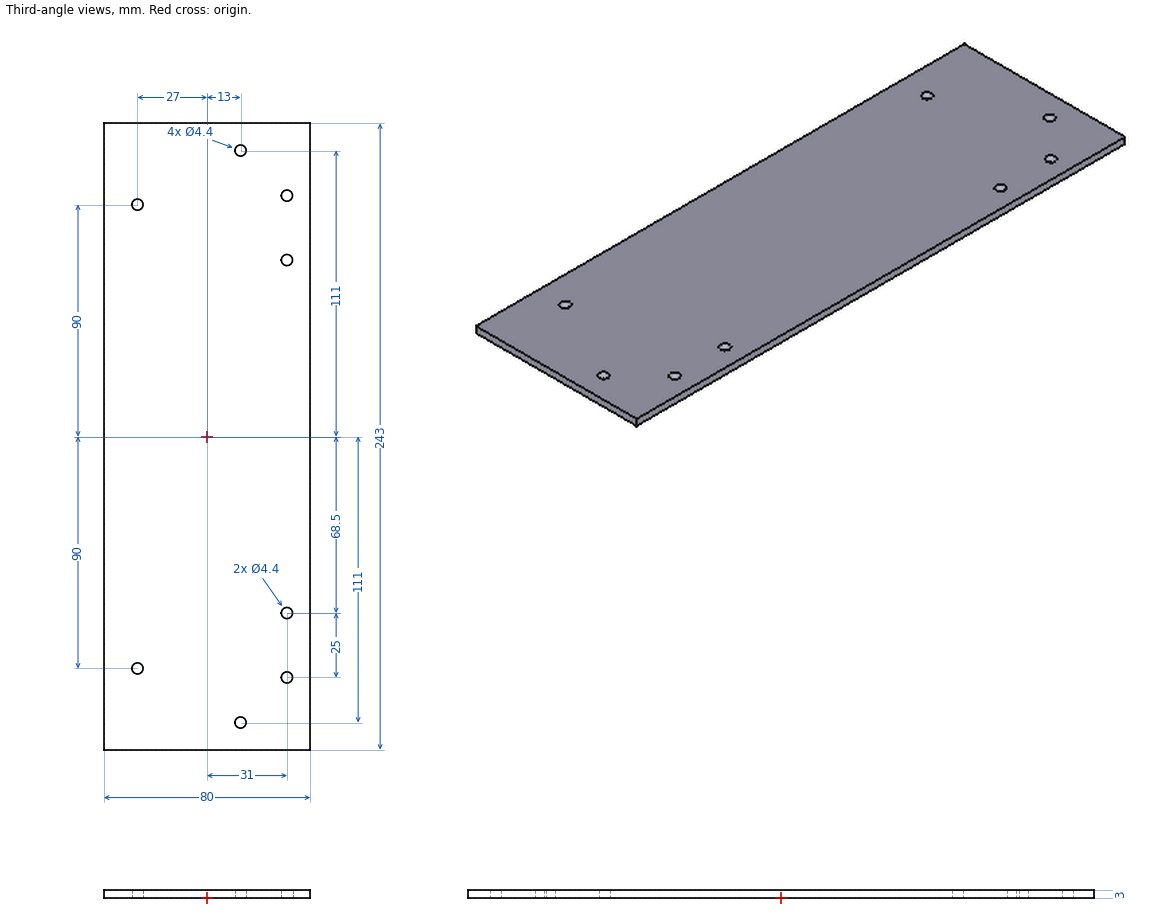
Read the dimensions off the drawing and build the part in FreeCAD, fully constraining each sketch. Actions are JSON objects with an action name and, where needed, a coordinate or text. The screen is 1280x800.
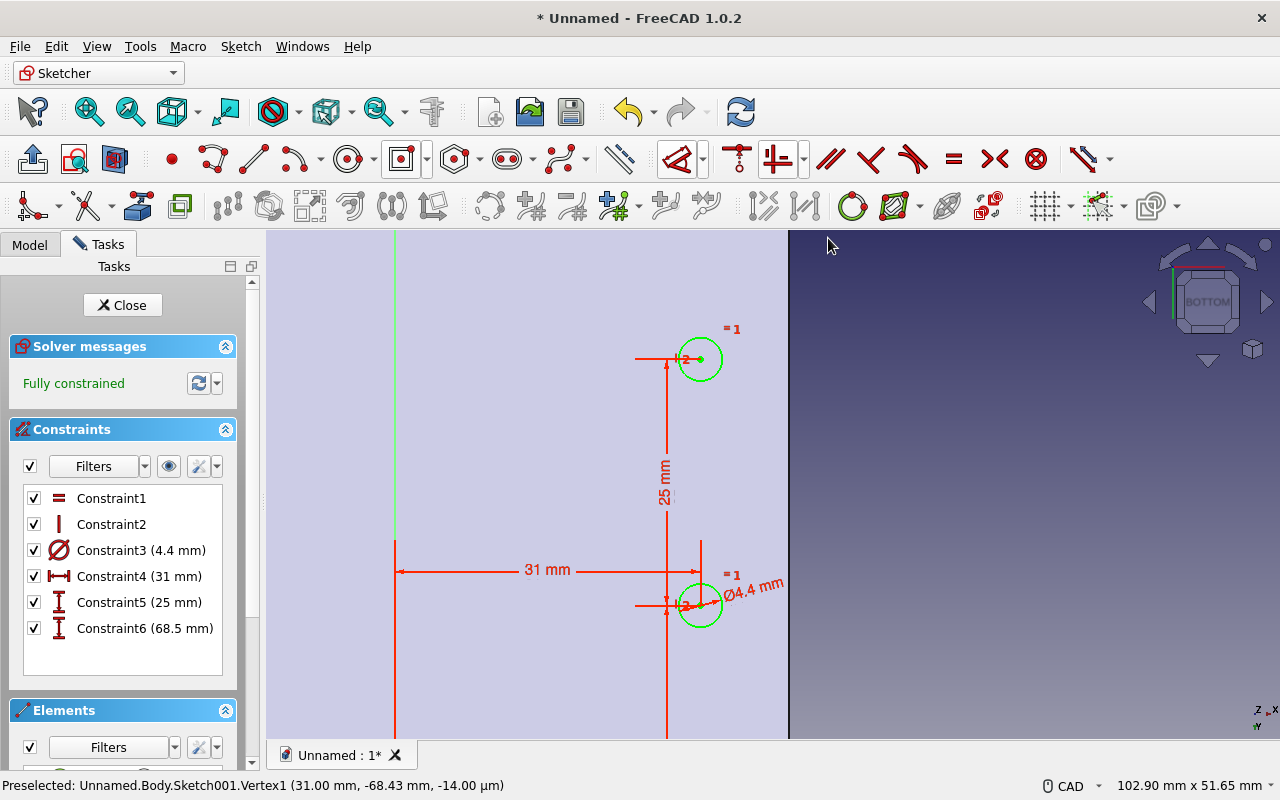
{"action": "left_click", "coordinate": [123, 305]}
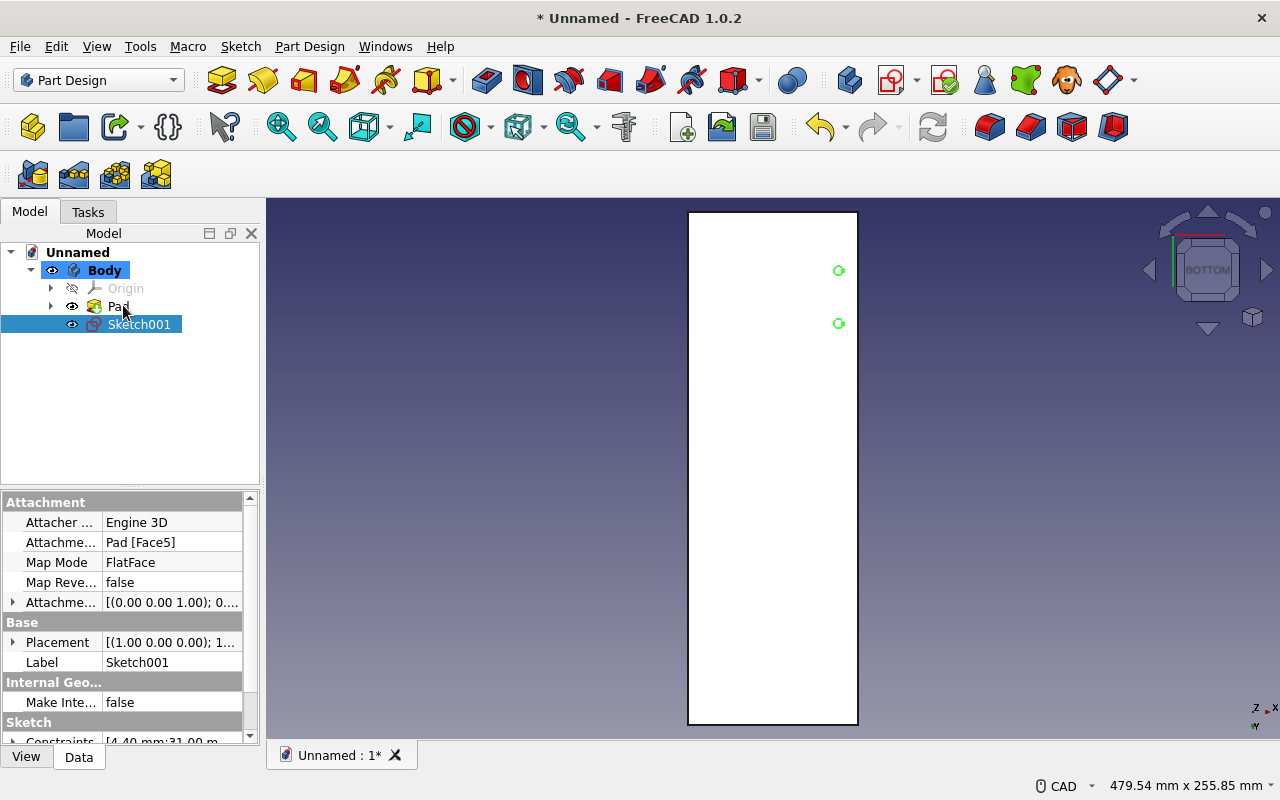
{"action": "left_click", "coordinate": [487, 80]}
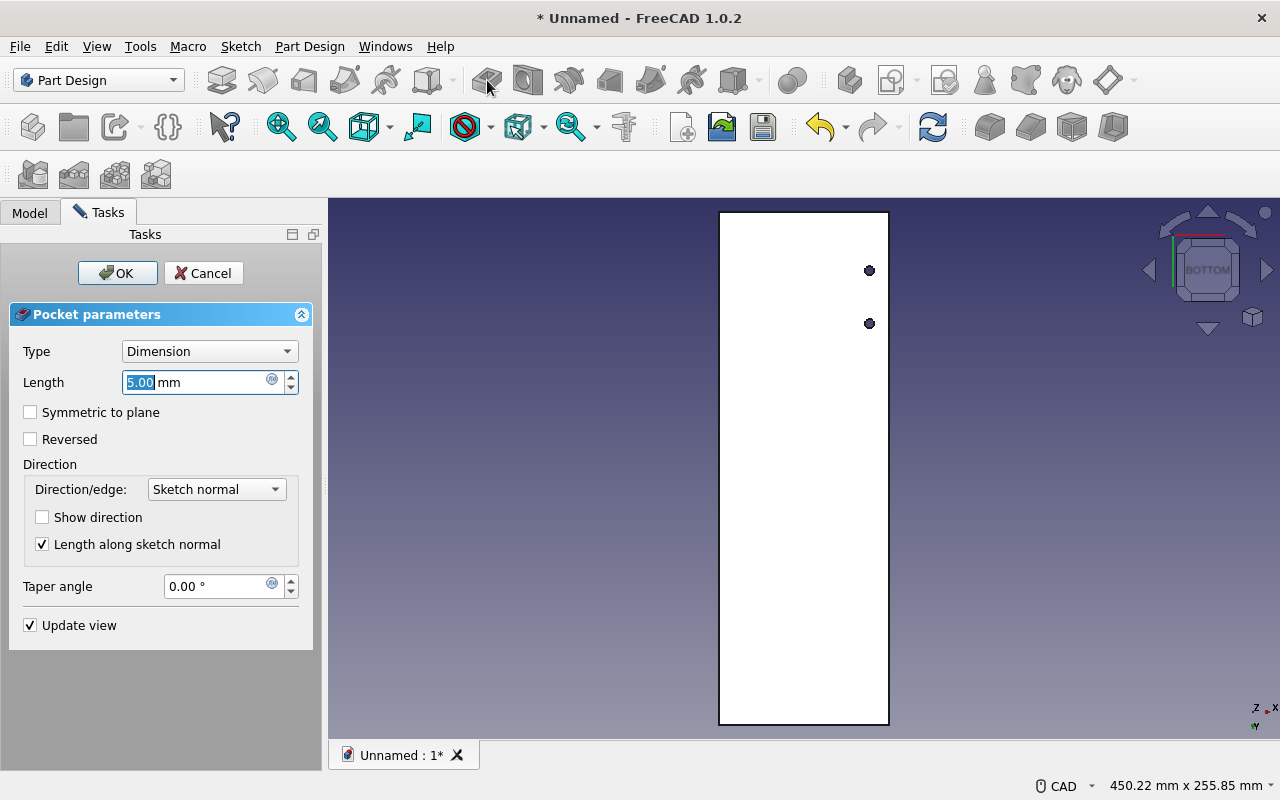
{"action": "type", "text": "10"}
{"action": "key", "text": "Tab"}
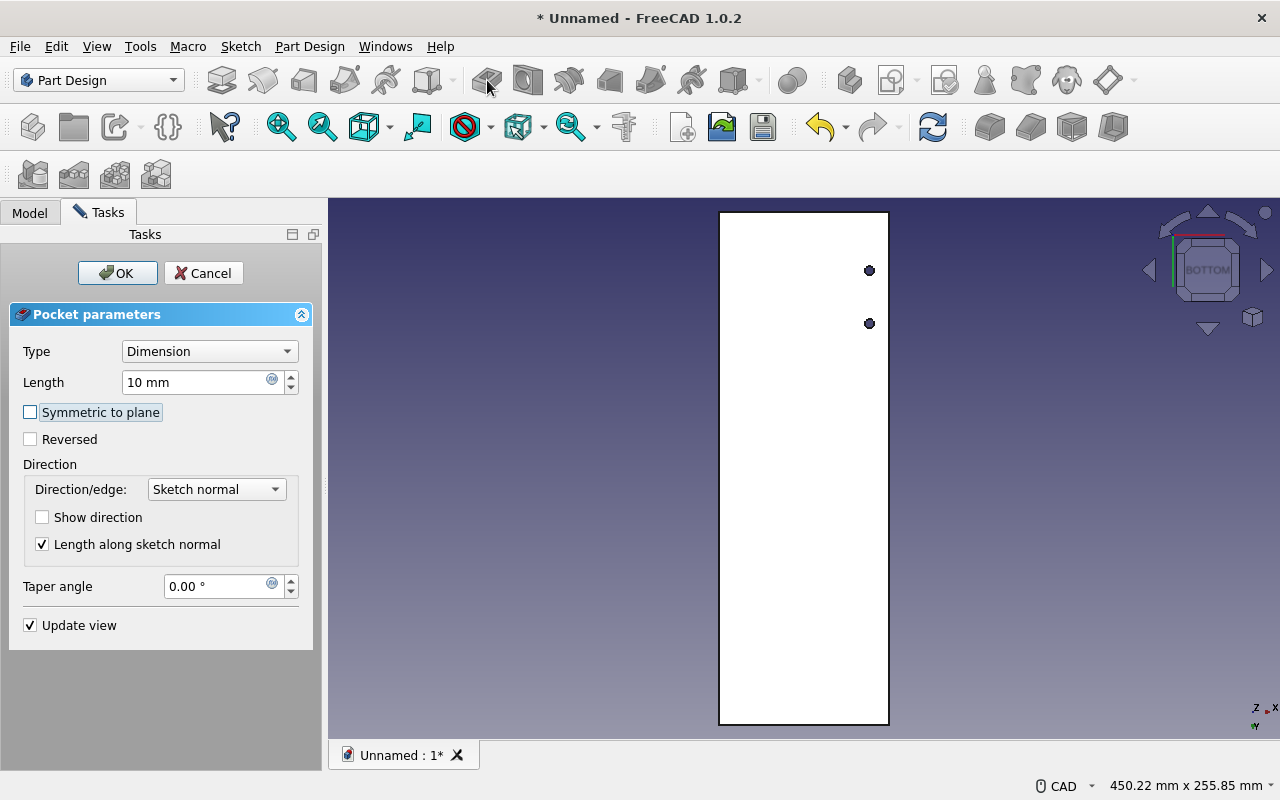
{"action": "left_click", "coordinate": [118, 273]}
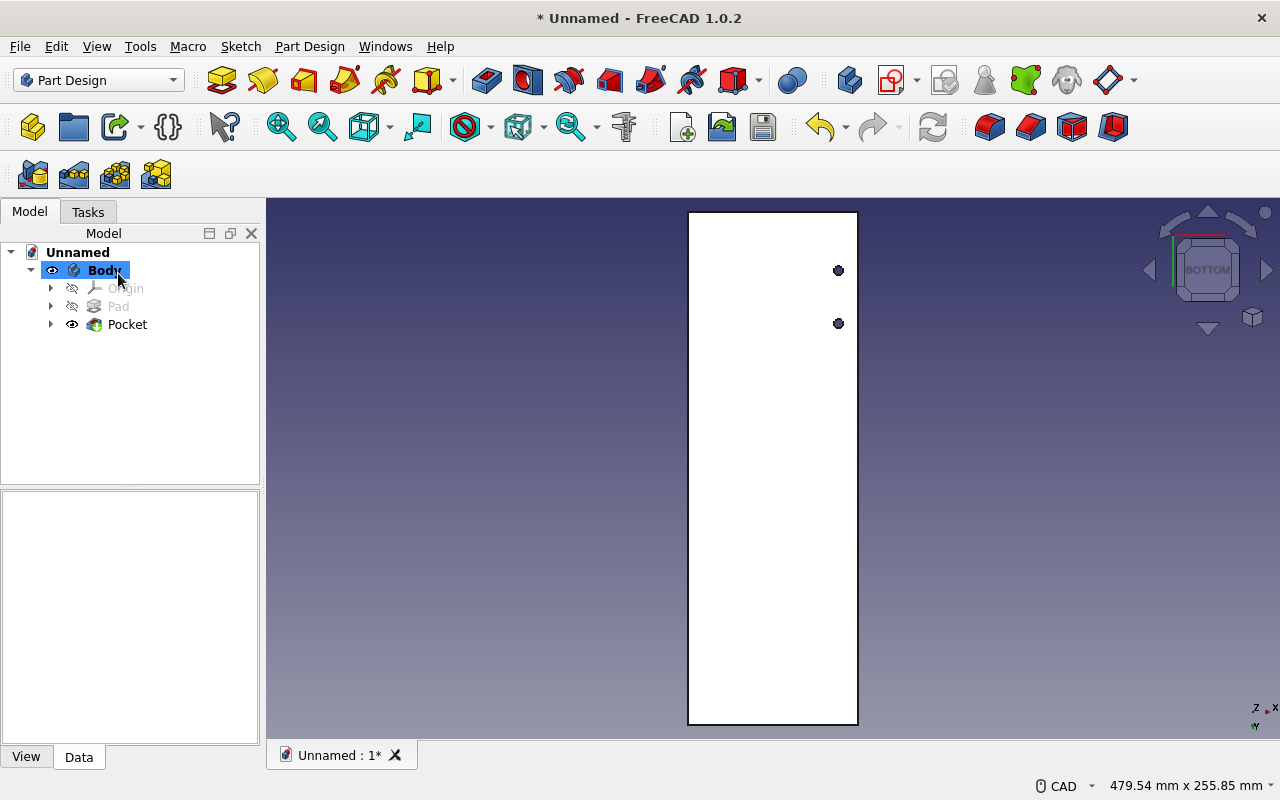
{"action": "left_click", "coordinate": [117, 324]}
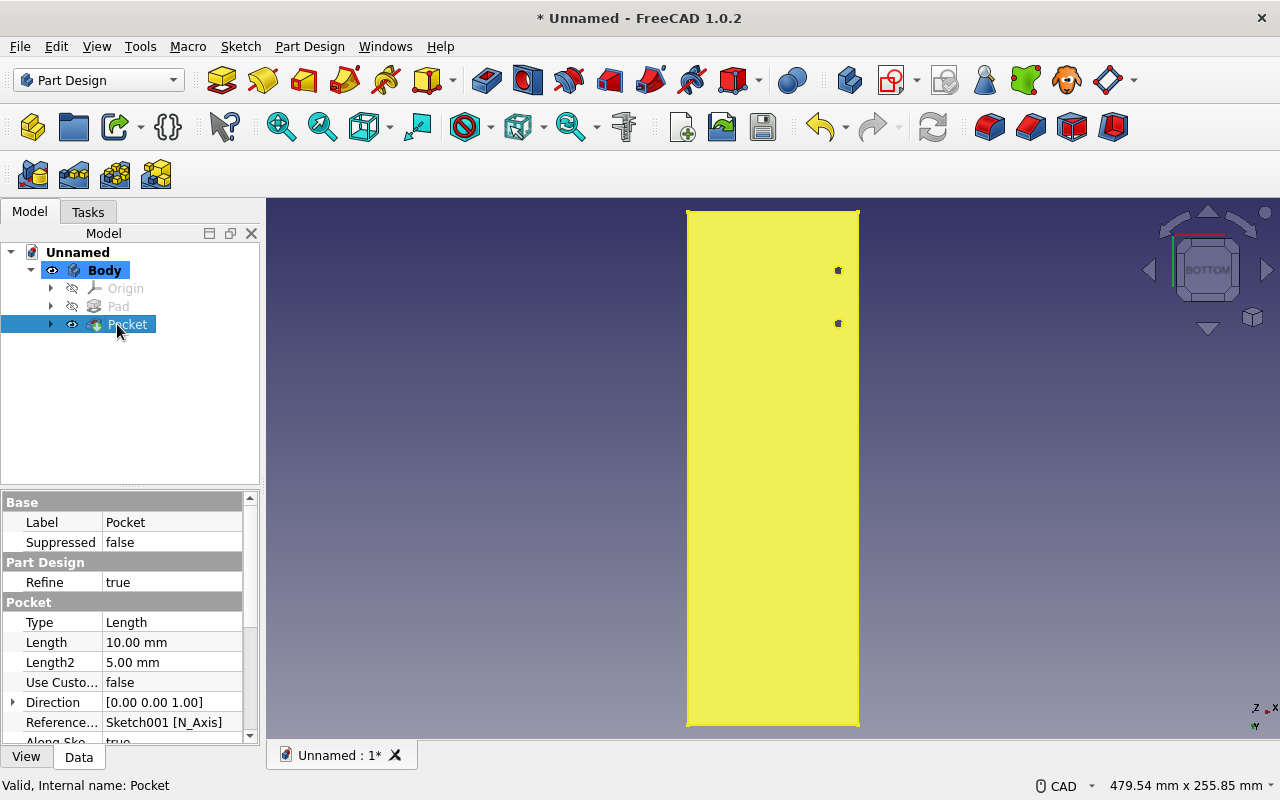
{"action": "left_click", "coordinate": [33, 174]}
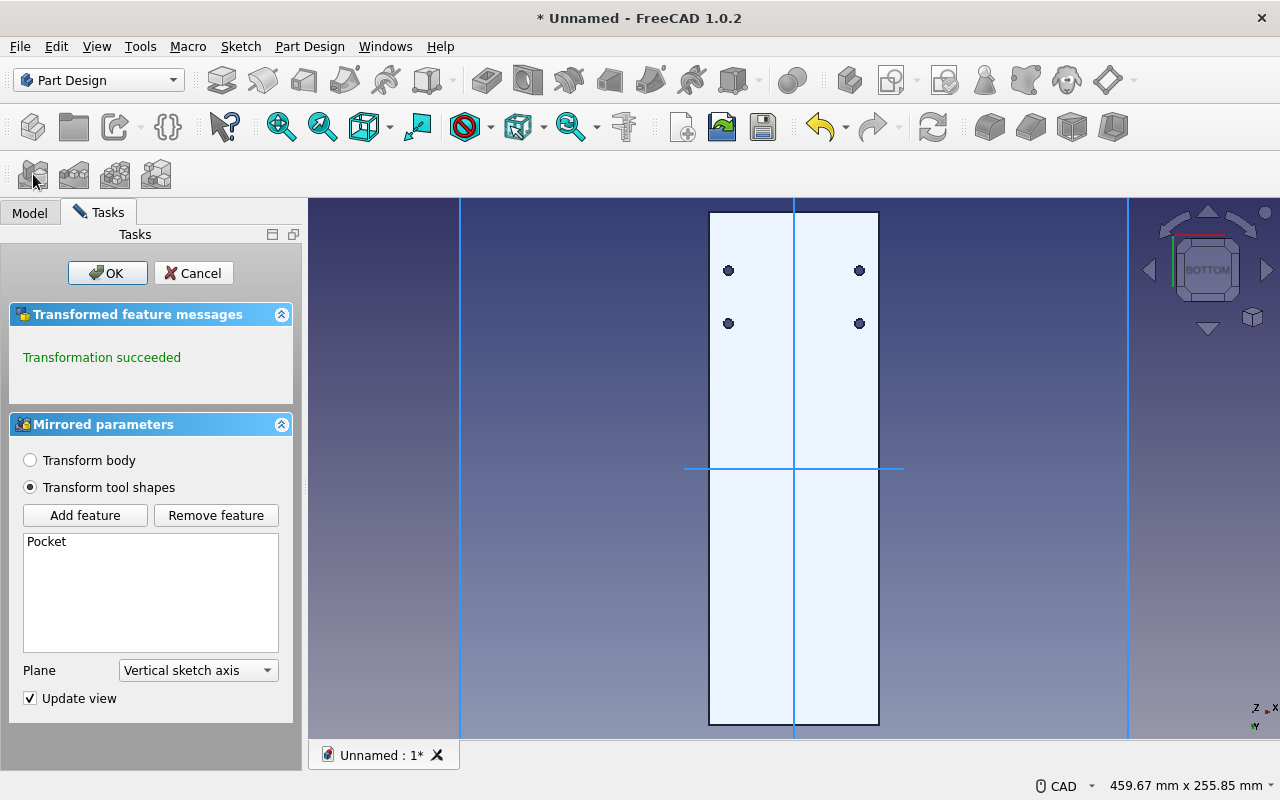
{"action": "left_click", "coordinate": [199, 670]}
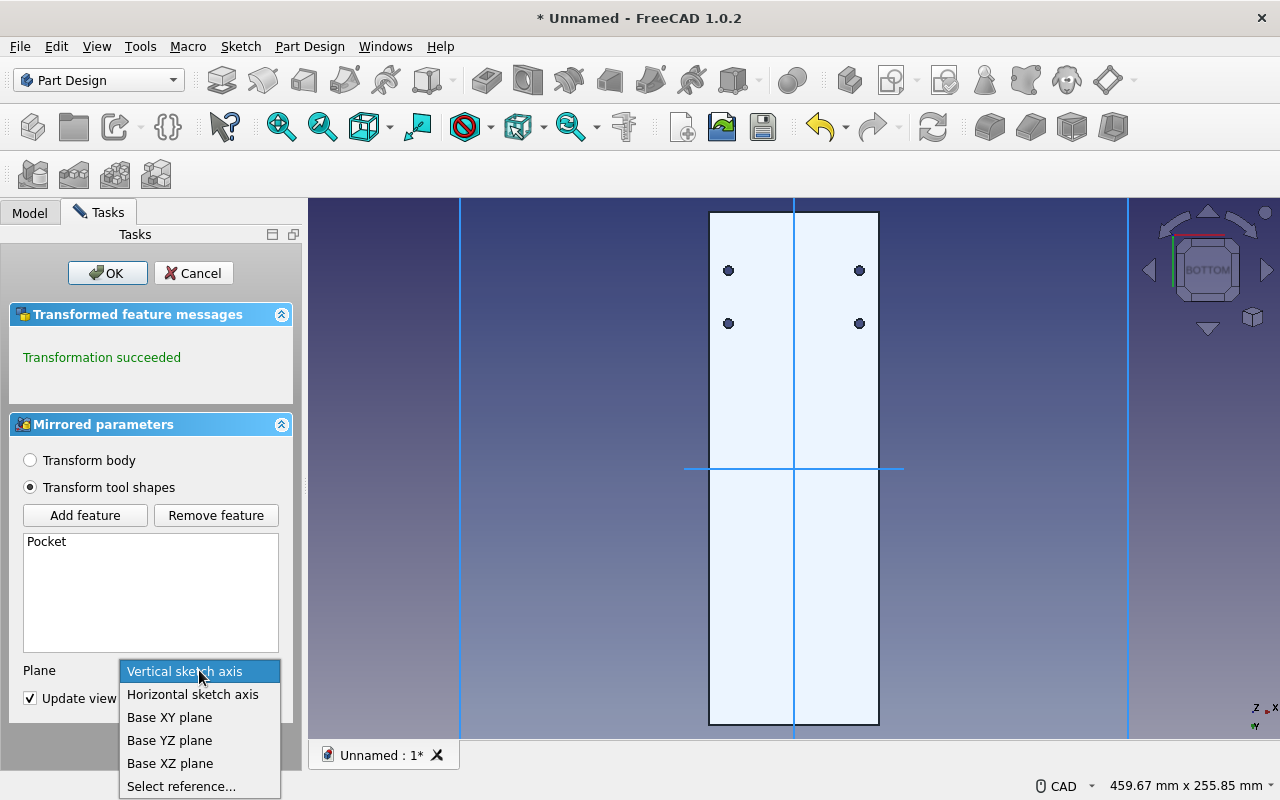
{"action": "left_click", "coordinate": [198, 764]}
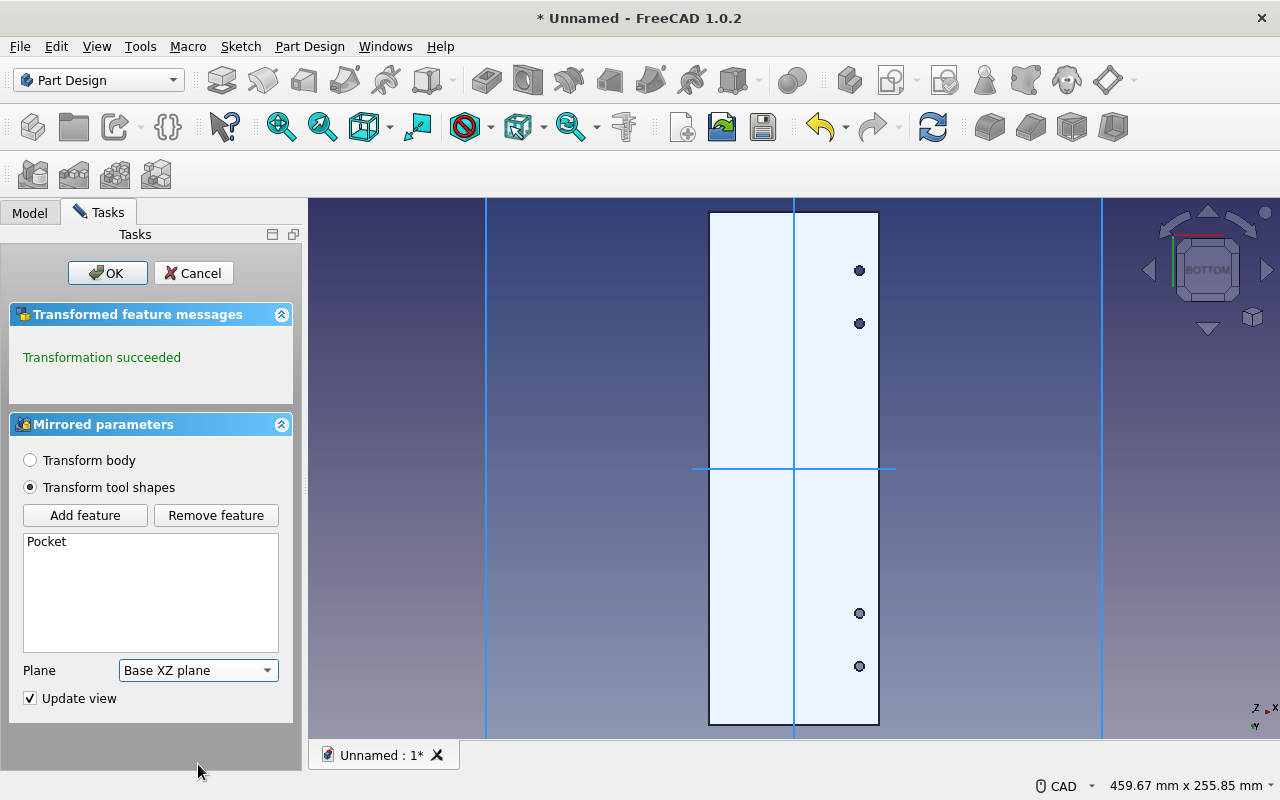
{"action": "left_click", "coordinate": [108, 273]}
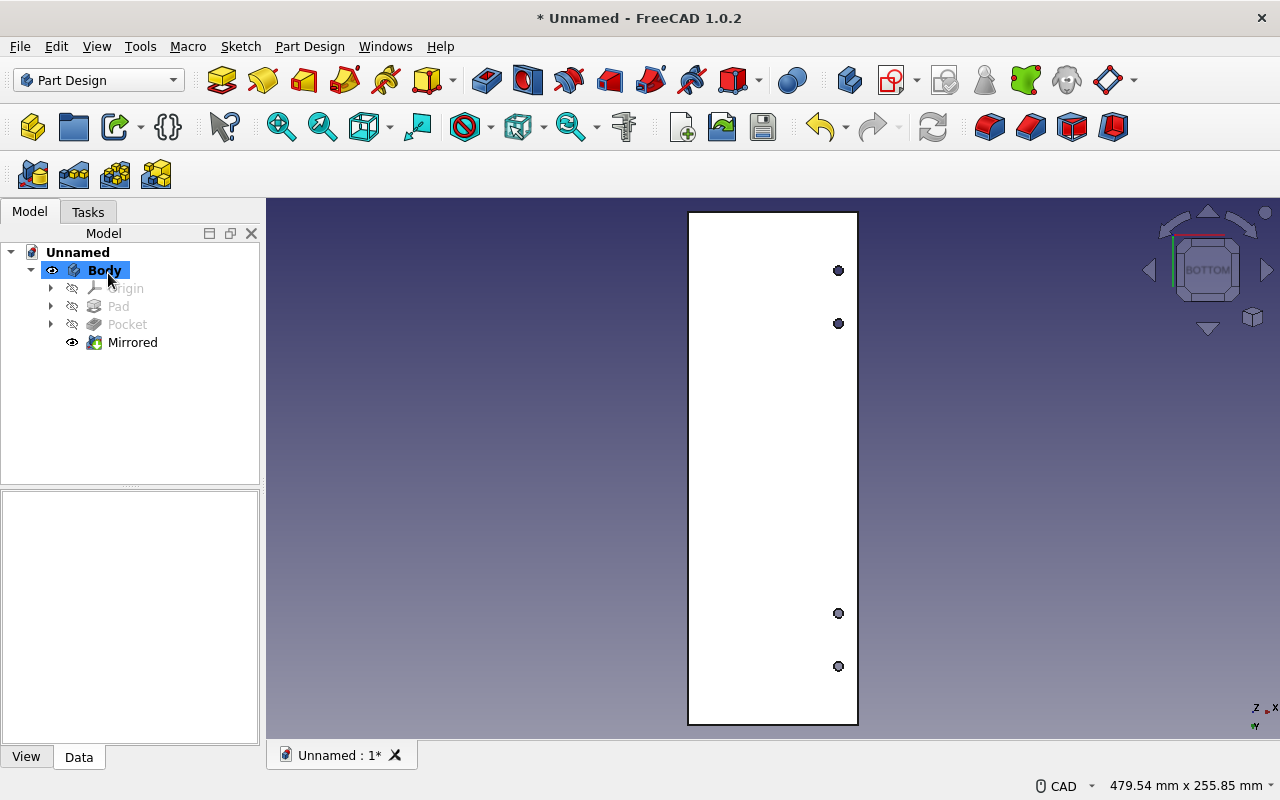
{"action": "left_click", "coordinate": [773, 541]}